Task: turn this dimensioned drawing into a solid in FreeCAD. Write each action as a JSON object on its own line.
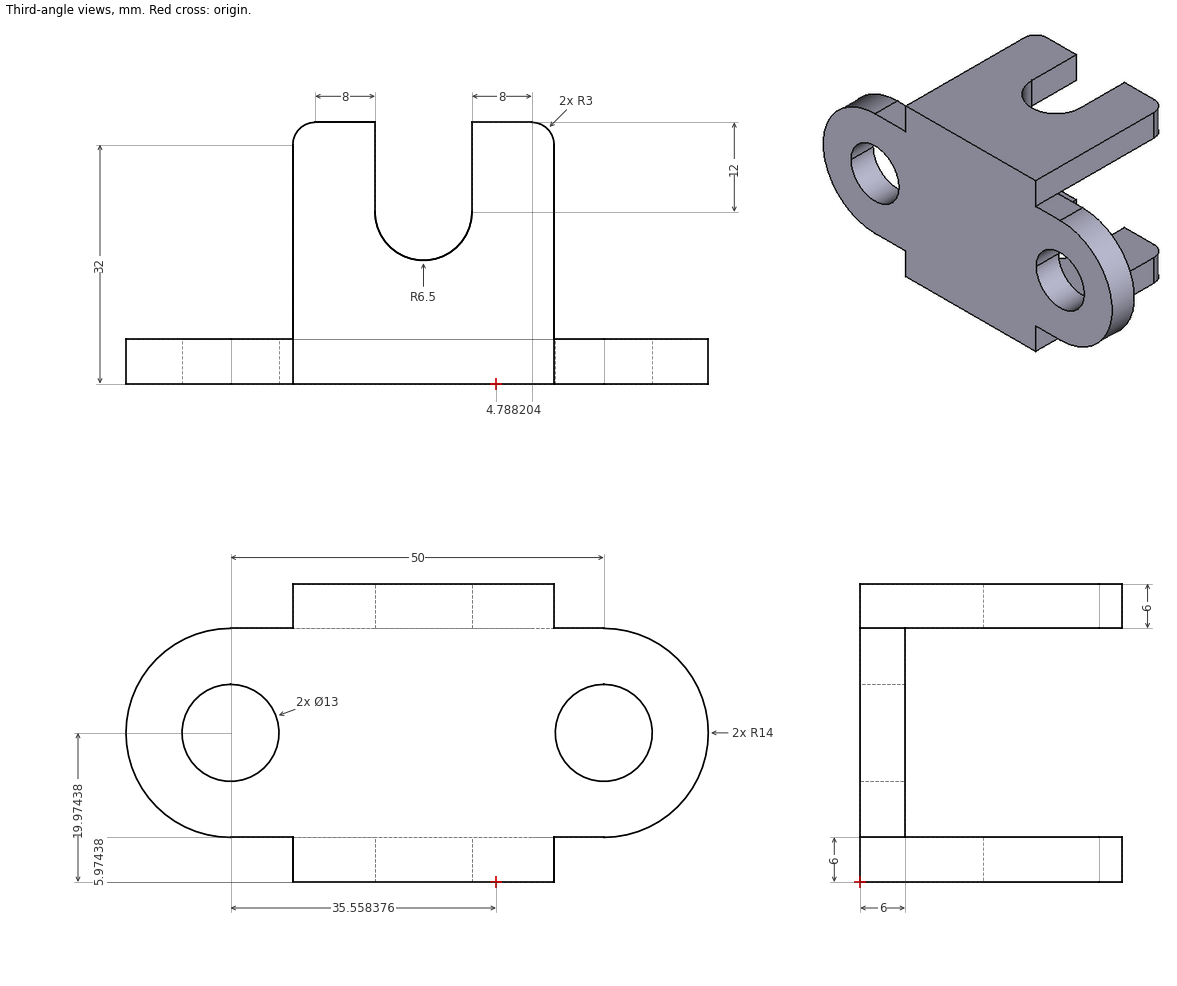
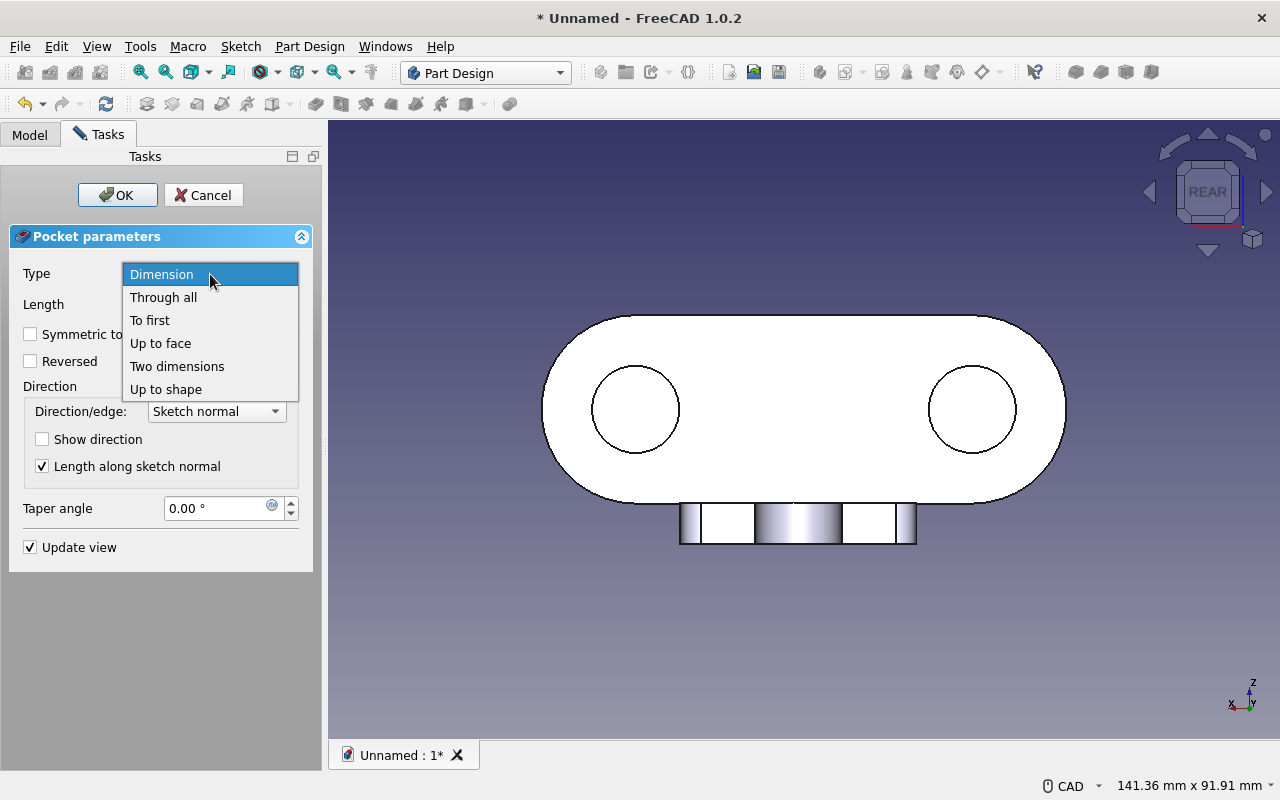
{"action": "left_click", "coordinate": [208, 298]}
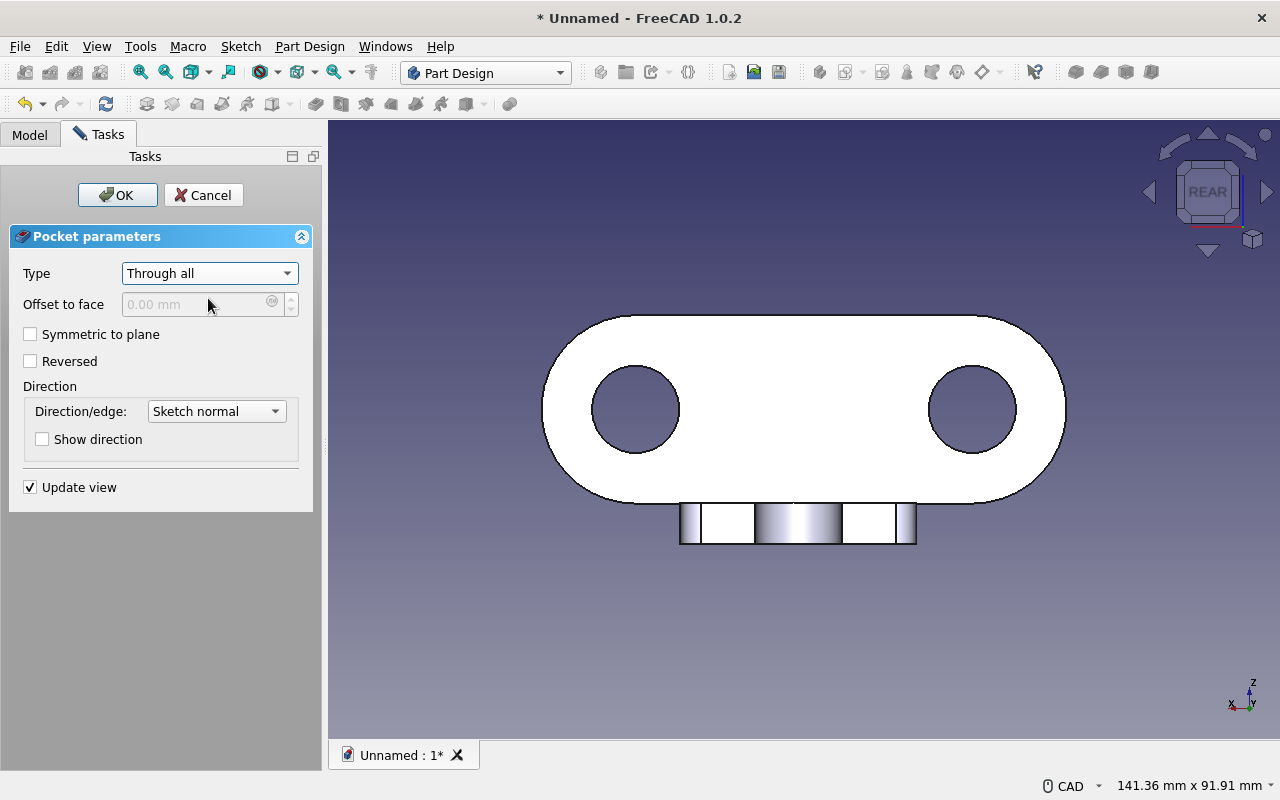
{"action": "left_click", "coordinate": [118, 195]}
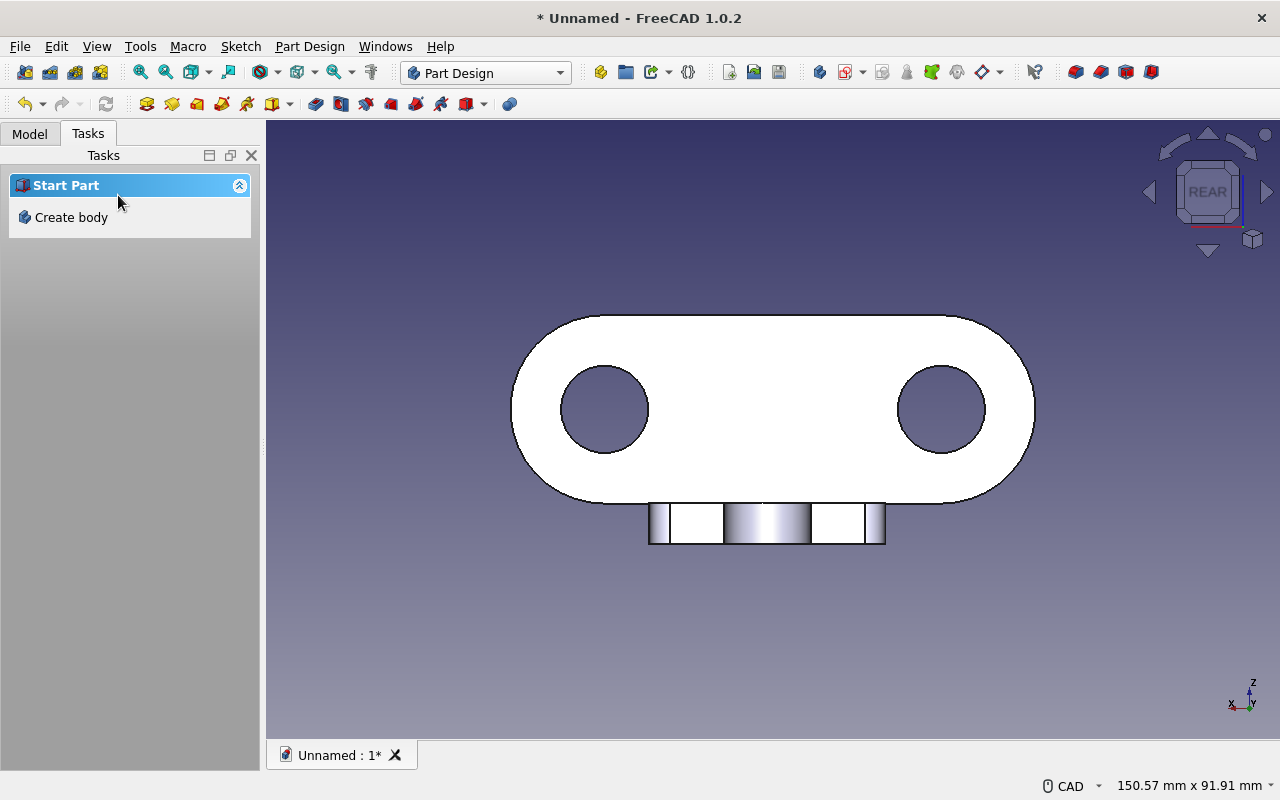
{"action": "key", "text": "0"}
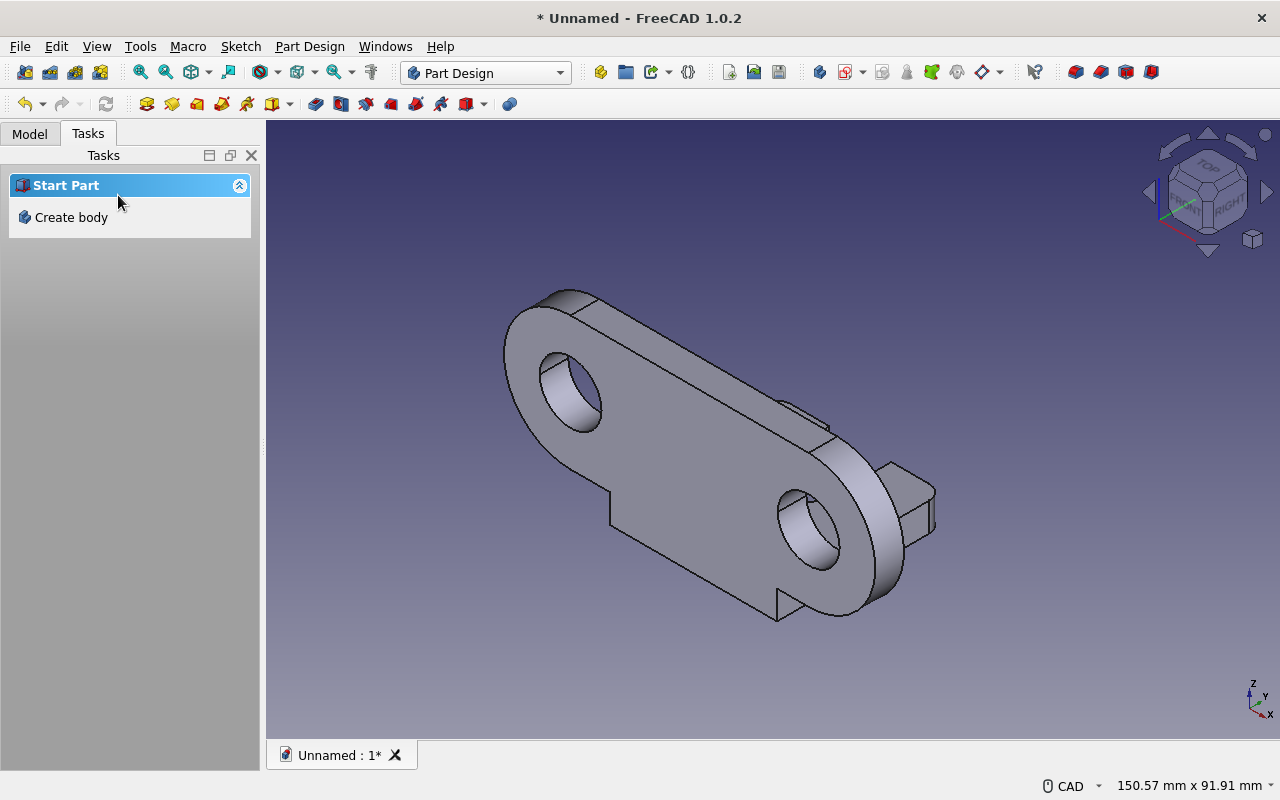
{"action": "left_click", "coordinate": [806, 434]}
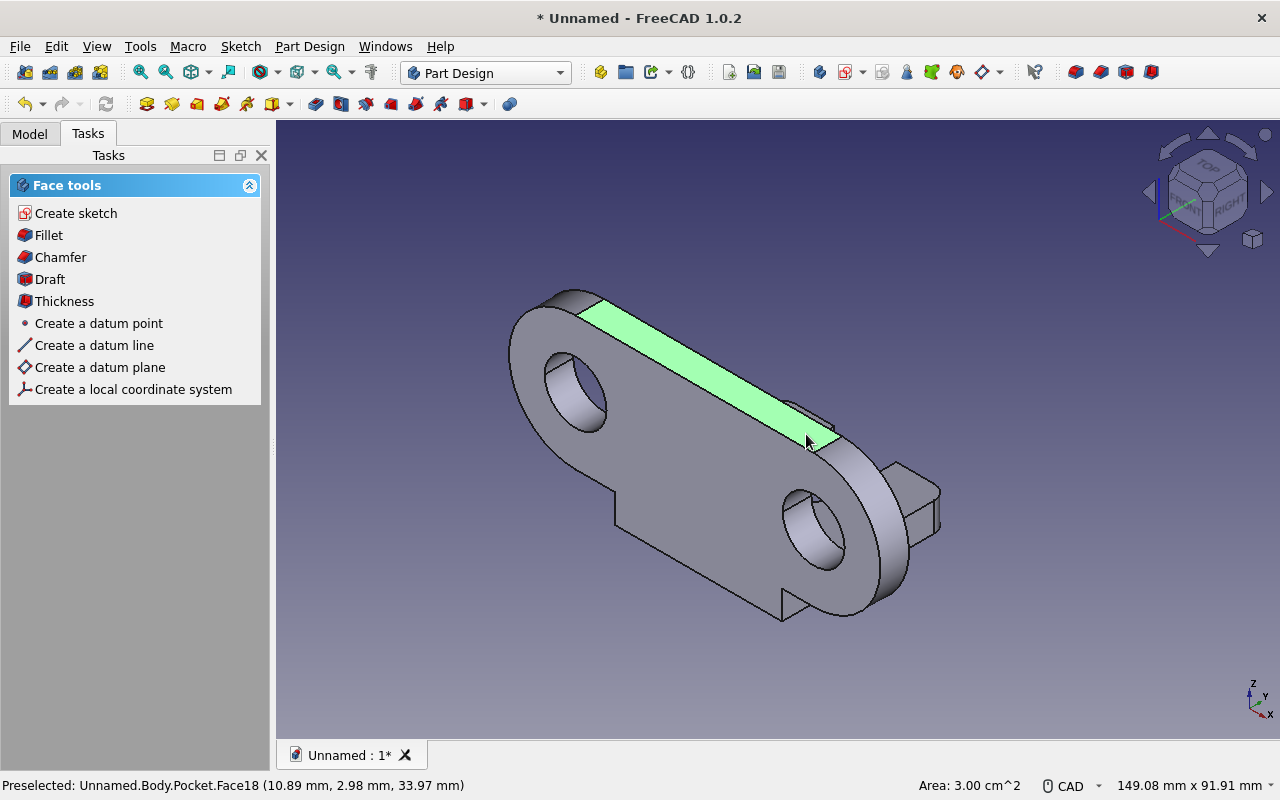
{"action": "left_click", "coordinate": [844, 72]}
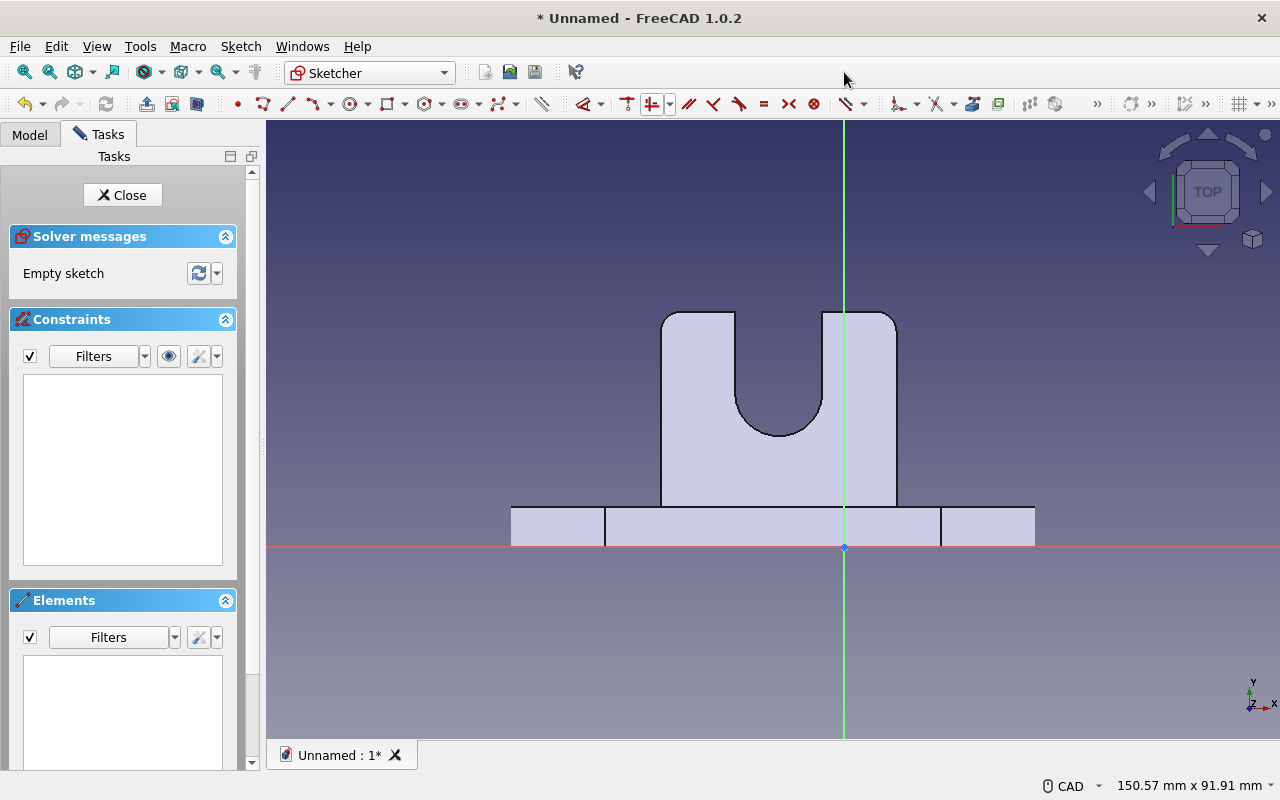
{"action": "scroll", "coordinate": [869, 429], "scroll_direction": "up", "scroll_amount": 3}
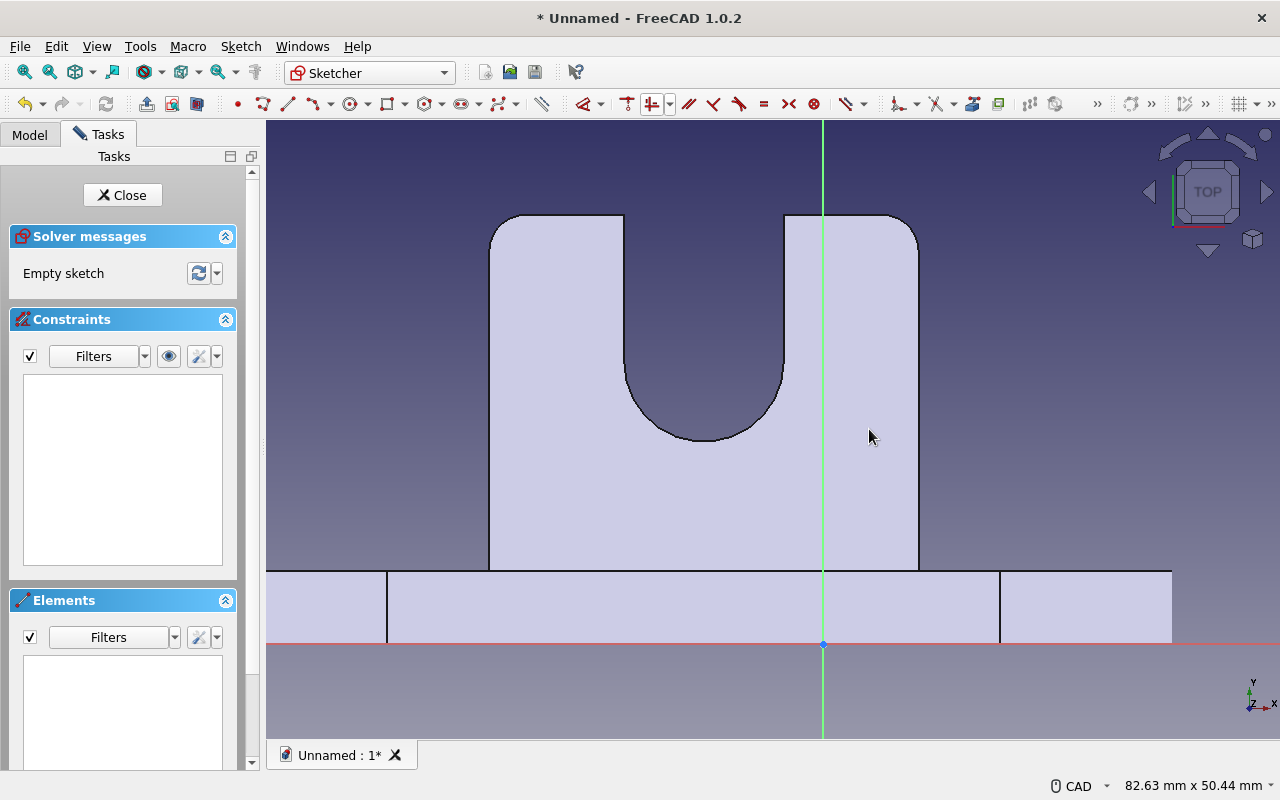
{"action": "left_click", "coordinate": [263, 104]}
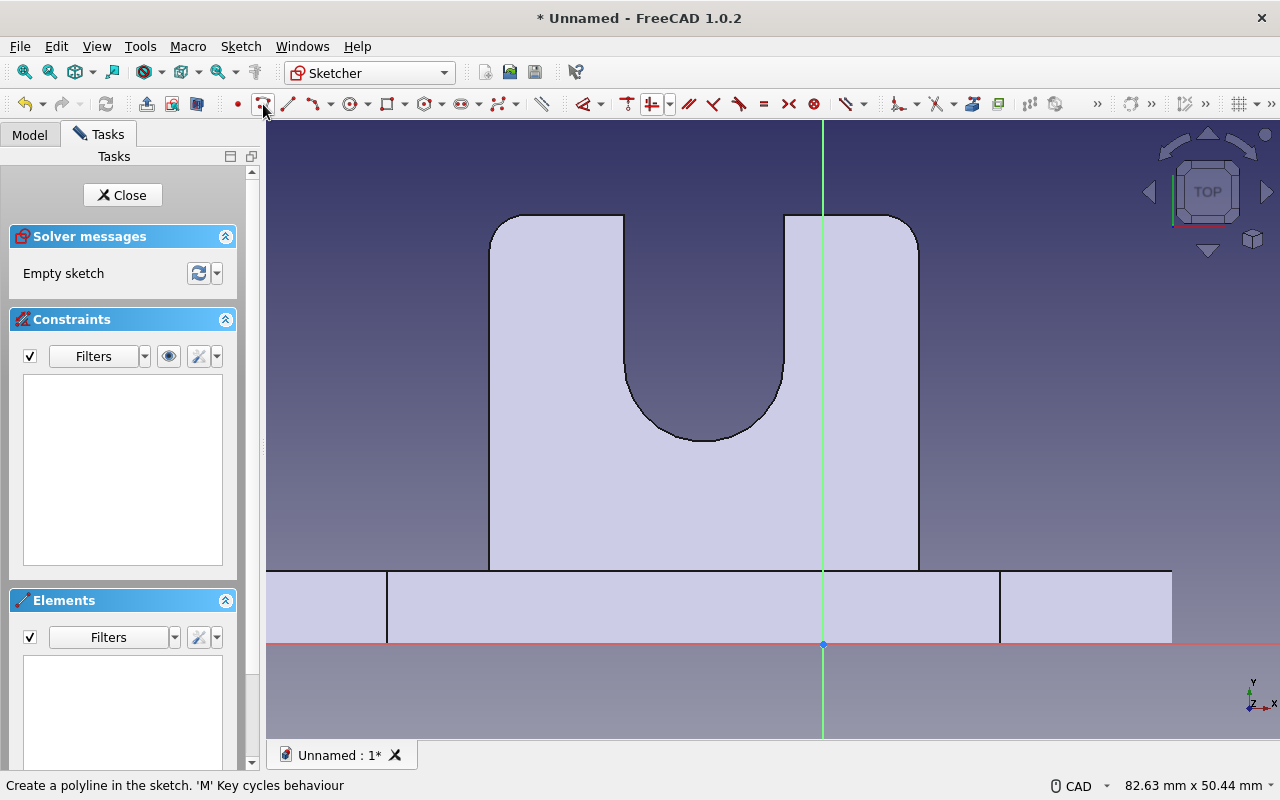
{"action": "left_click", "coordinate": [882, 215]}
{"action": "left_click", "coordinate": [784, 215]}
{"action": "left_click", "coordinate": [784, 362]}
{"action": "right_click", "coordinate": [784, 362]}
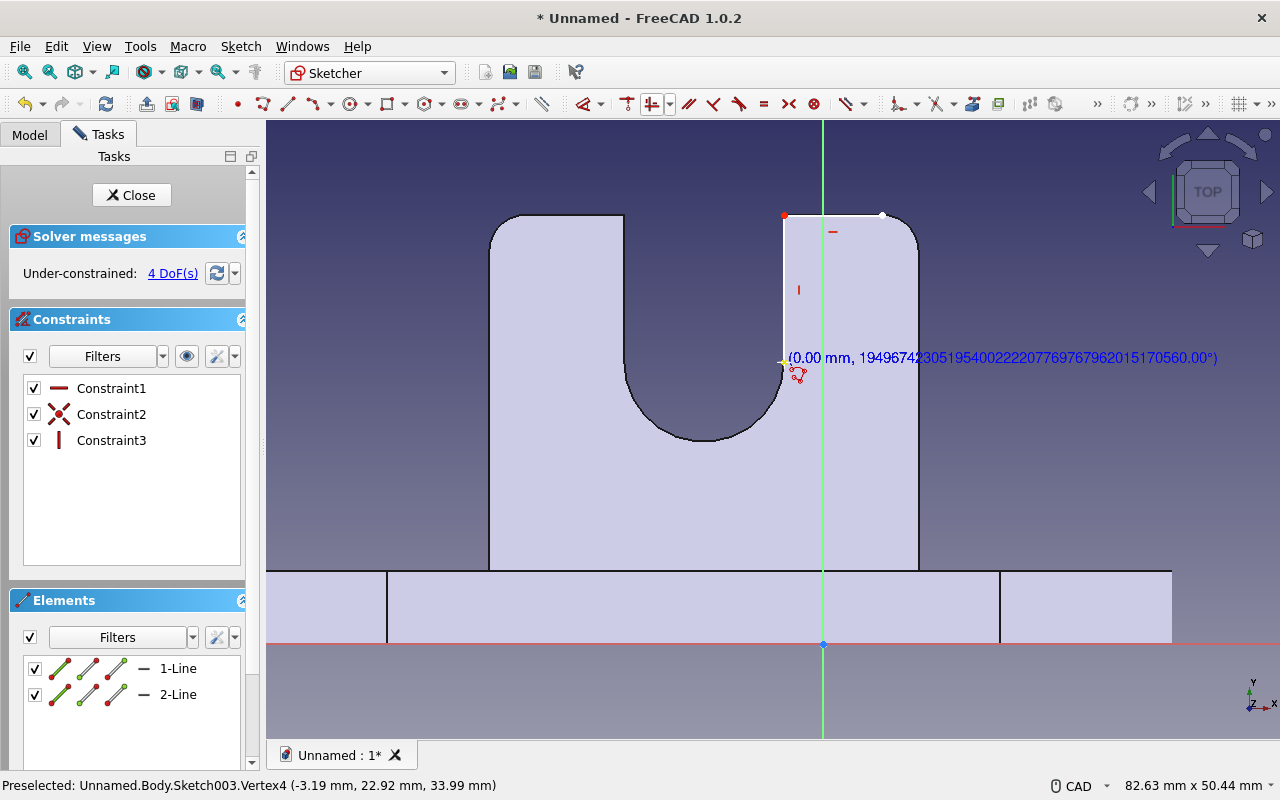
{"action": "left_click", "coordinate": [624, 362]}
{"action": "left_click", "coordinate": [624, 215]}
{"action": "left_click", "coordinate": [526, 215]}
{"action": "right_click", "coordinate": [526, 215]}